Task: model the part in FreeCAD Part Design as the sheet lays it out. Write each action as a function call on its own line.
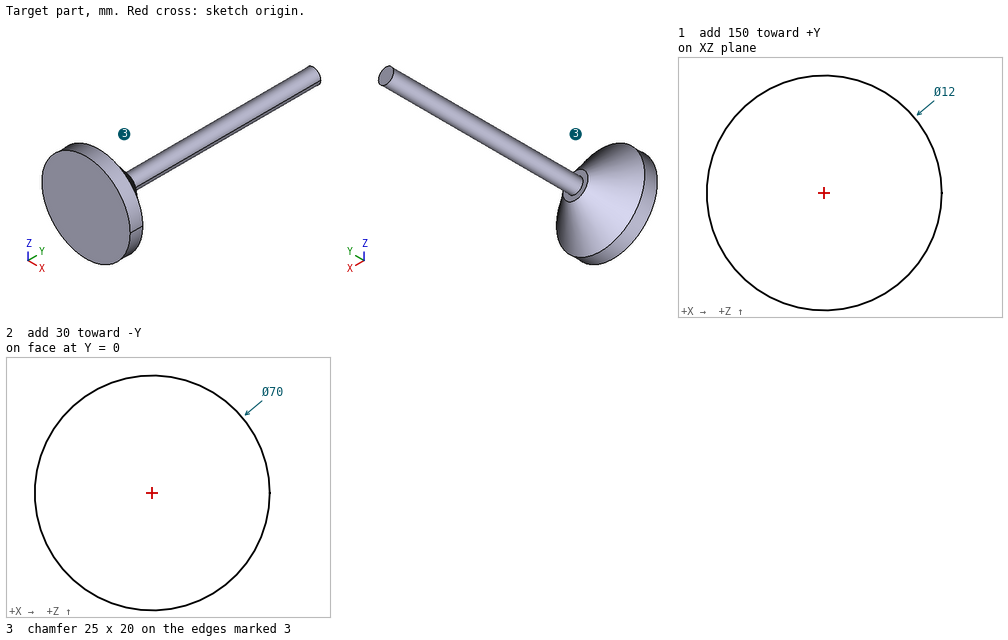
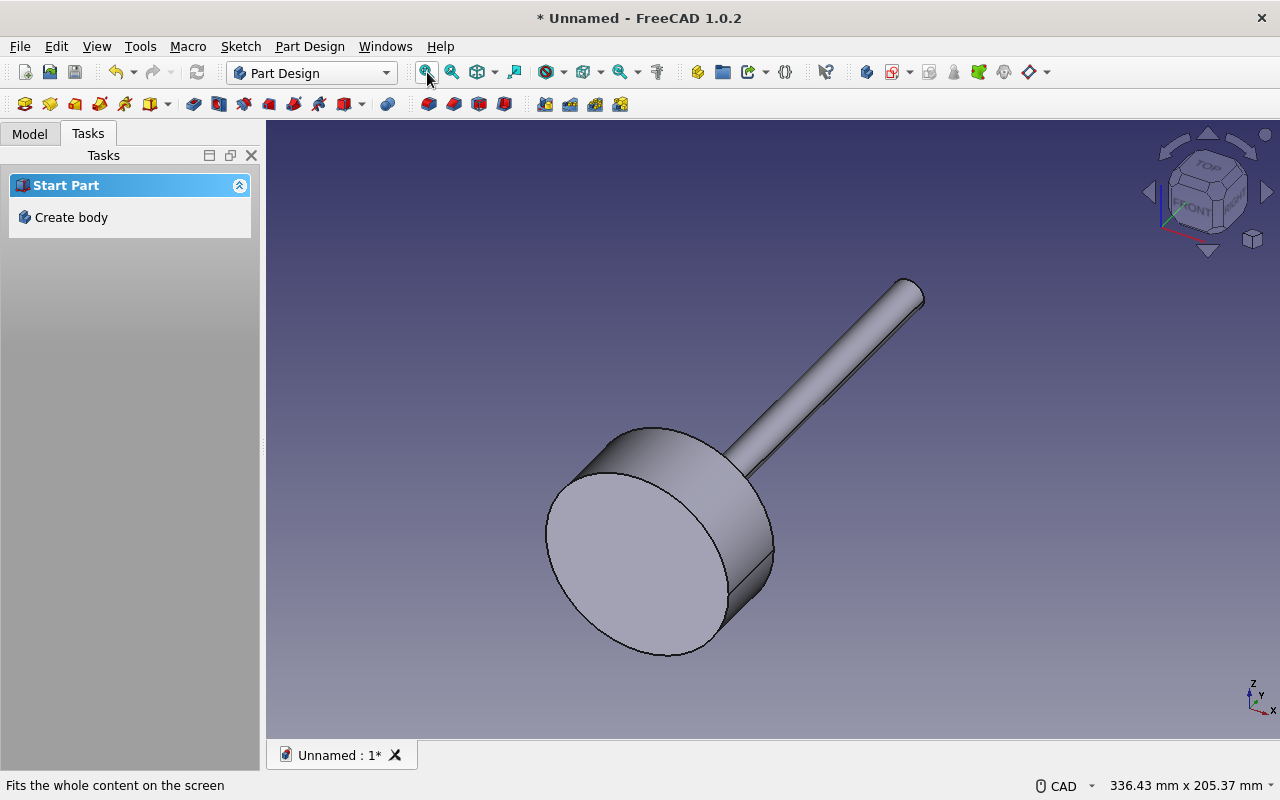
click(711, 445)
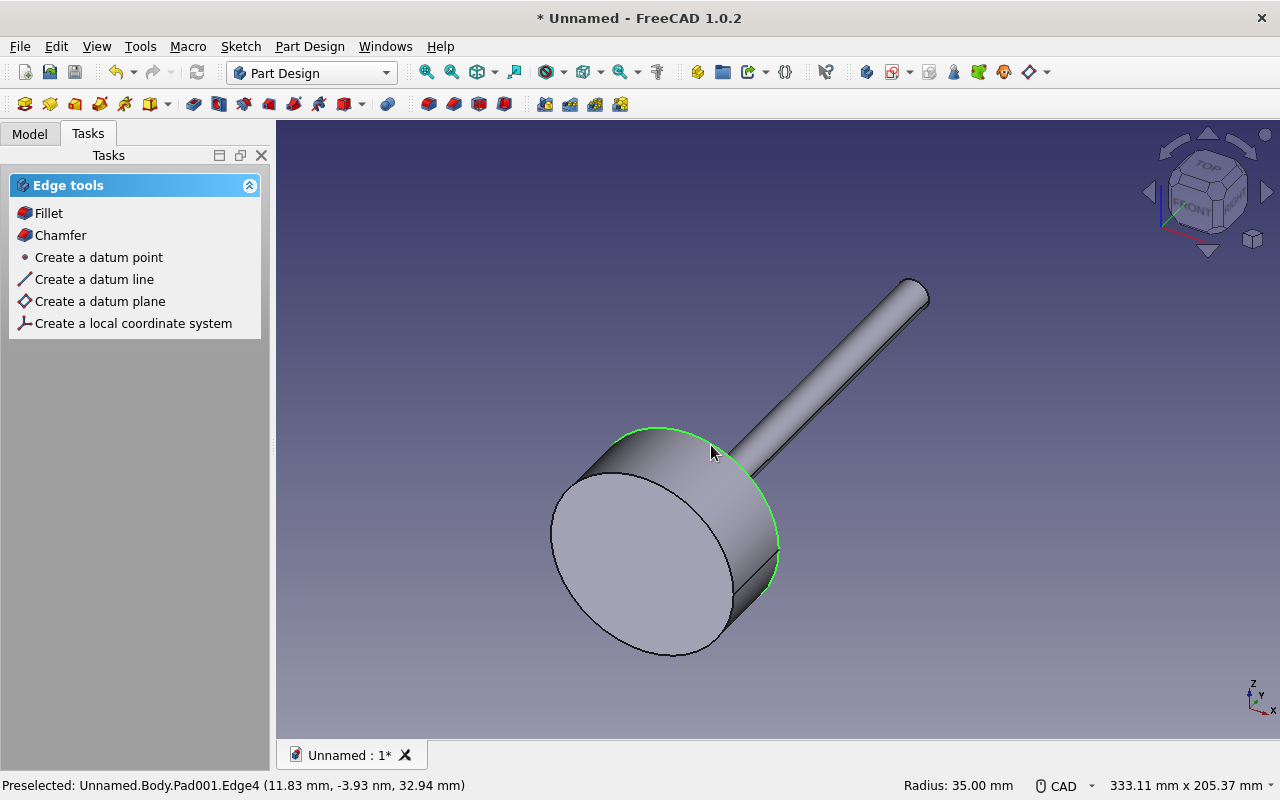
click(454, 104)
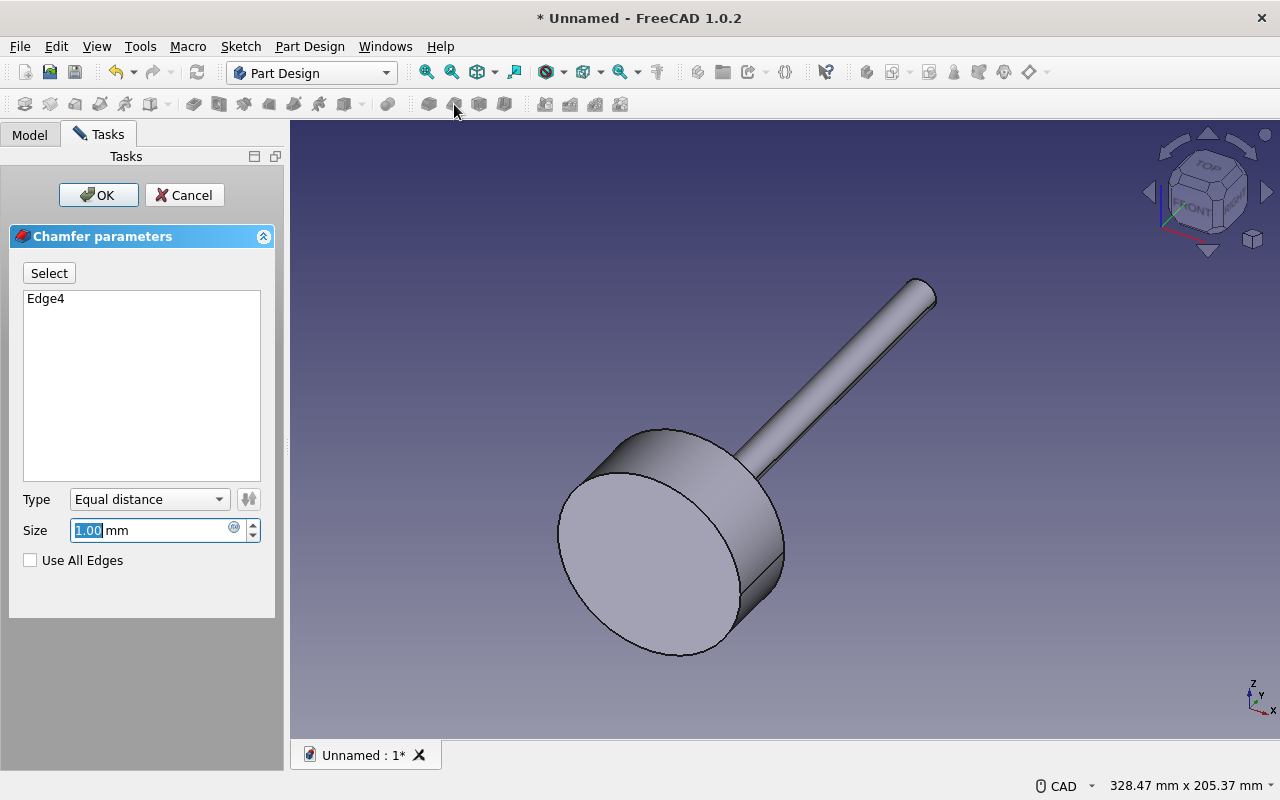
text(25)
key(Tab)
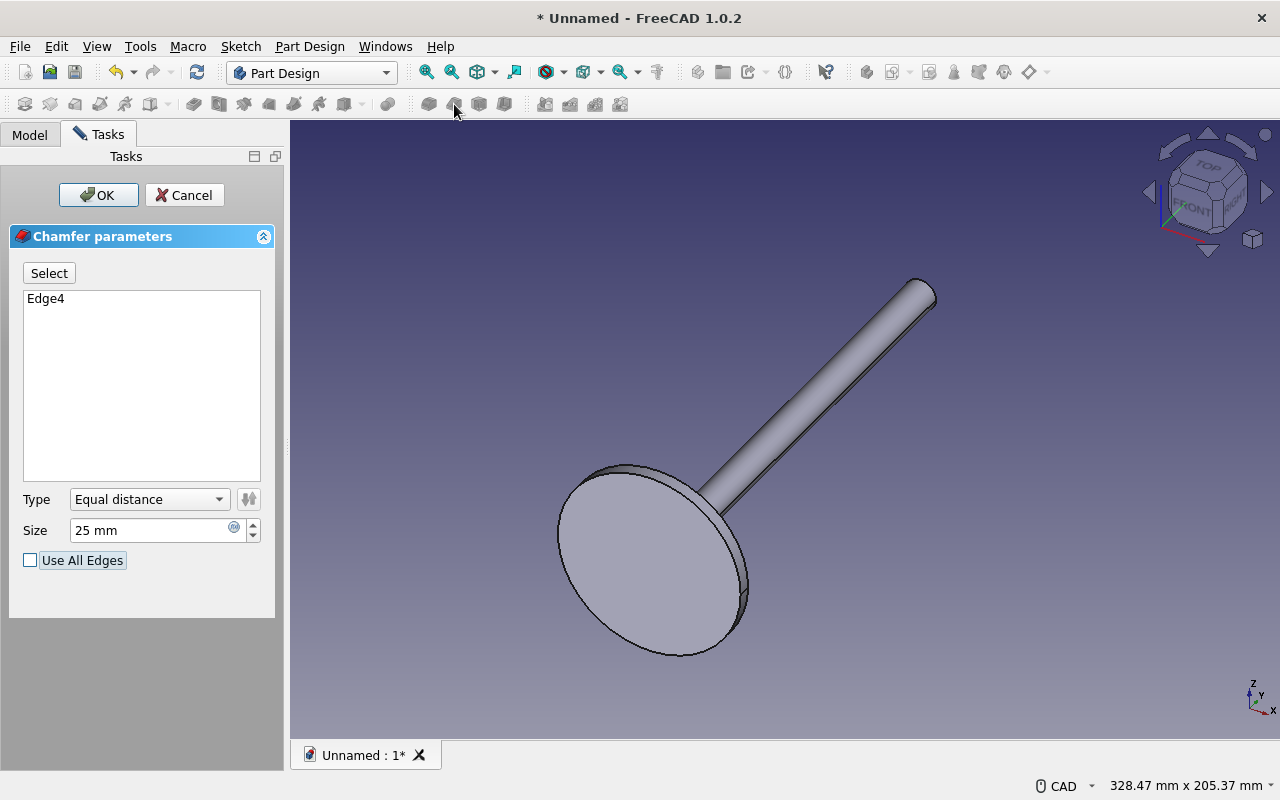
click(150, 500)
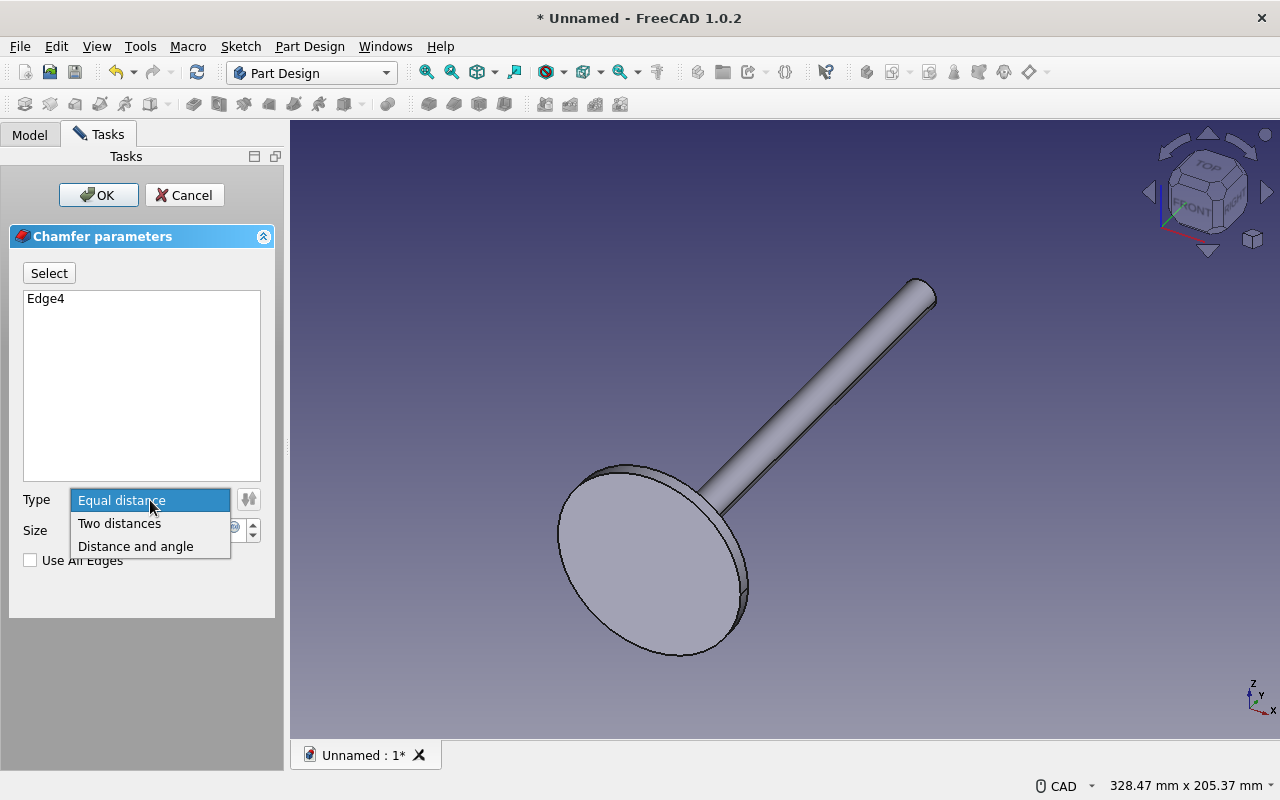
click(148, 524)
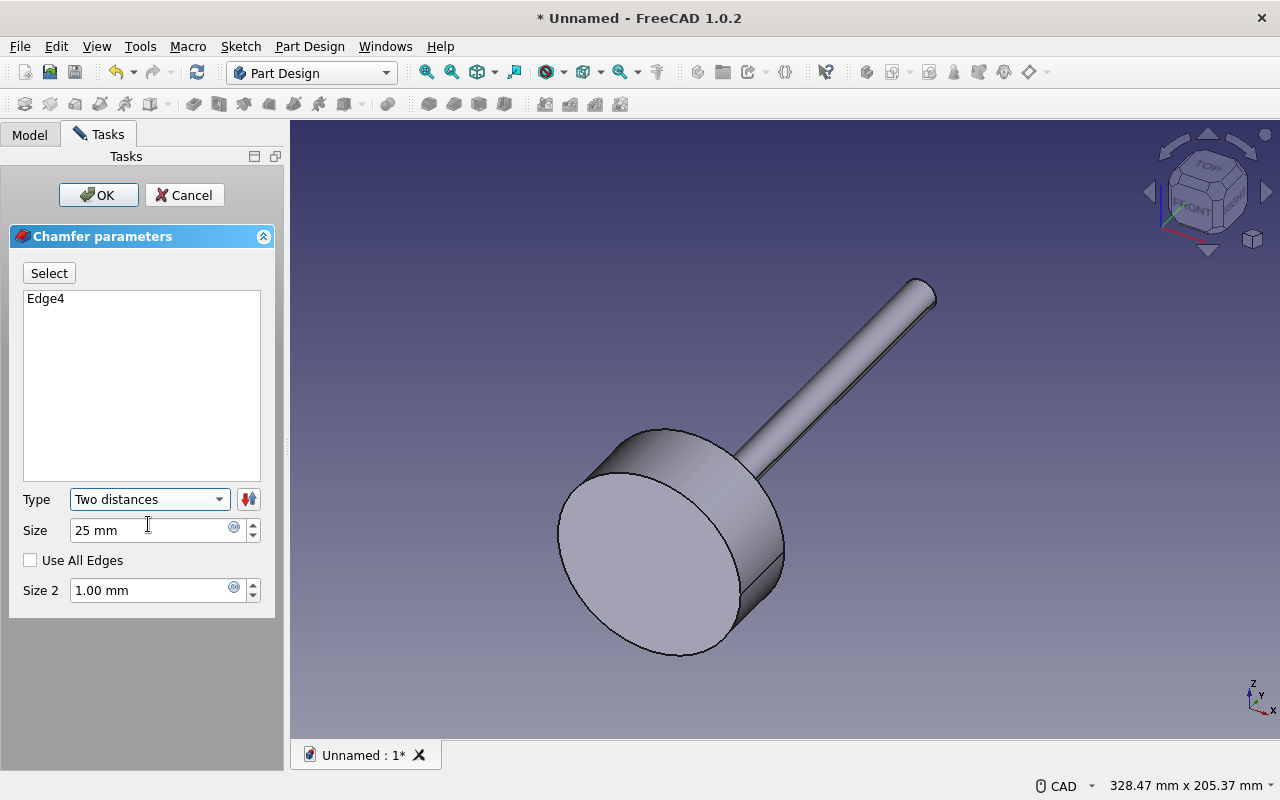
triple_click(158, 590)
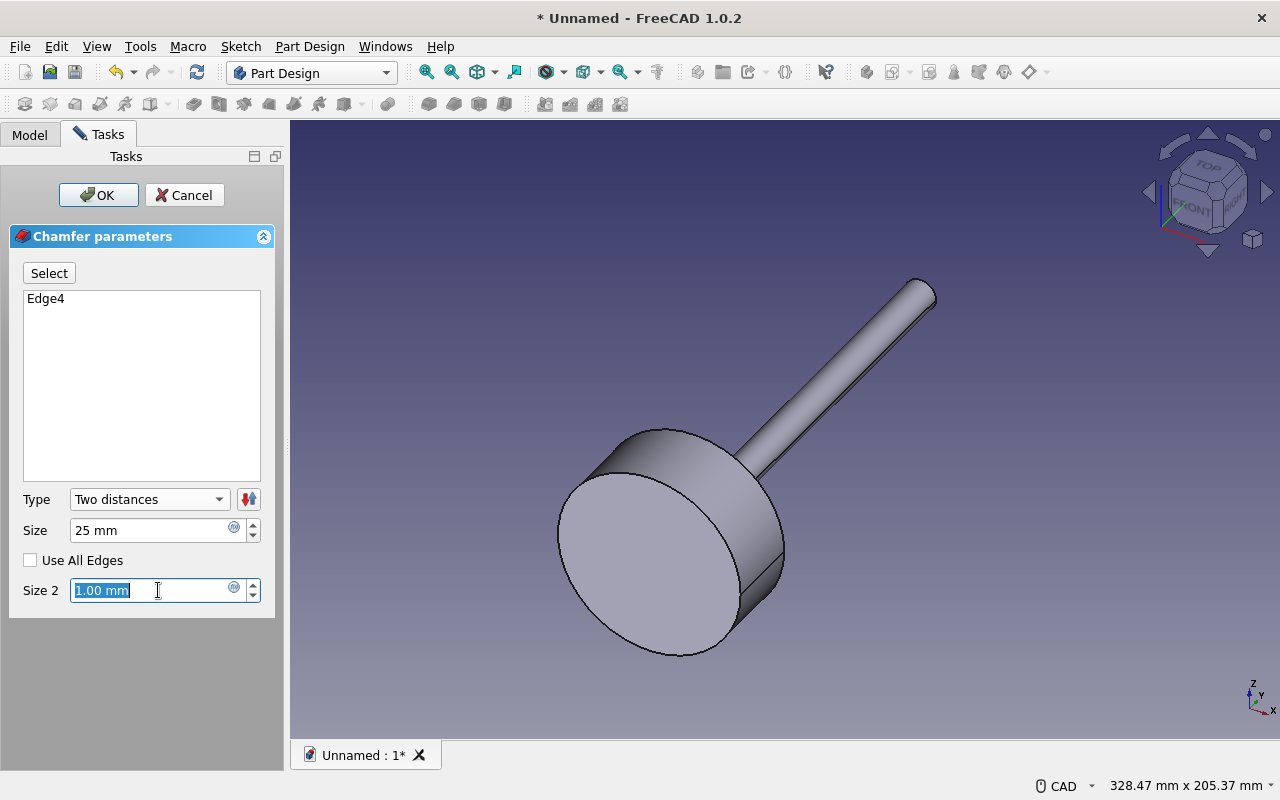
text(20)
key(Tab)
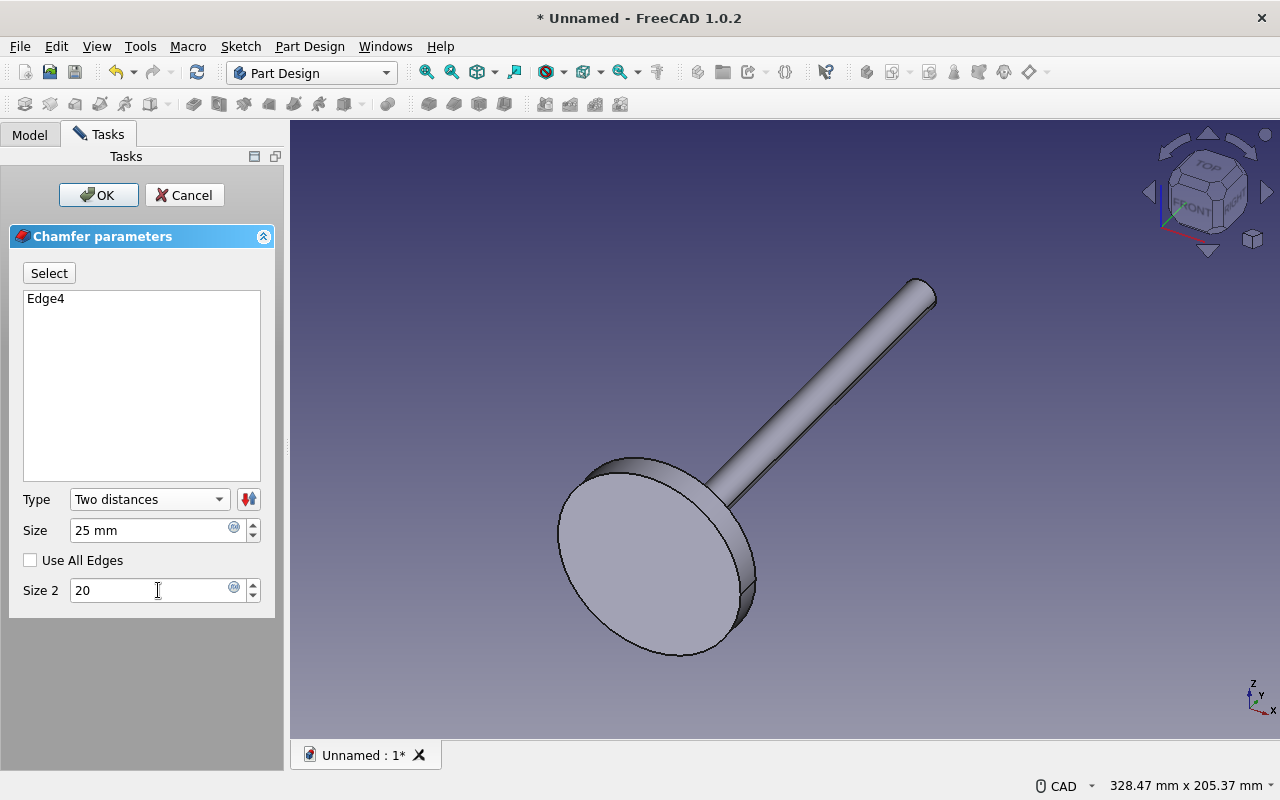
click(99, 195)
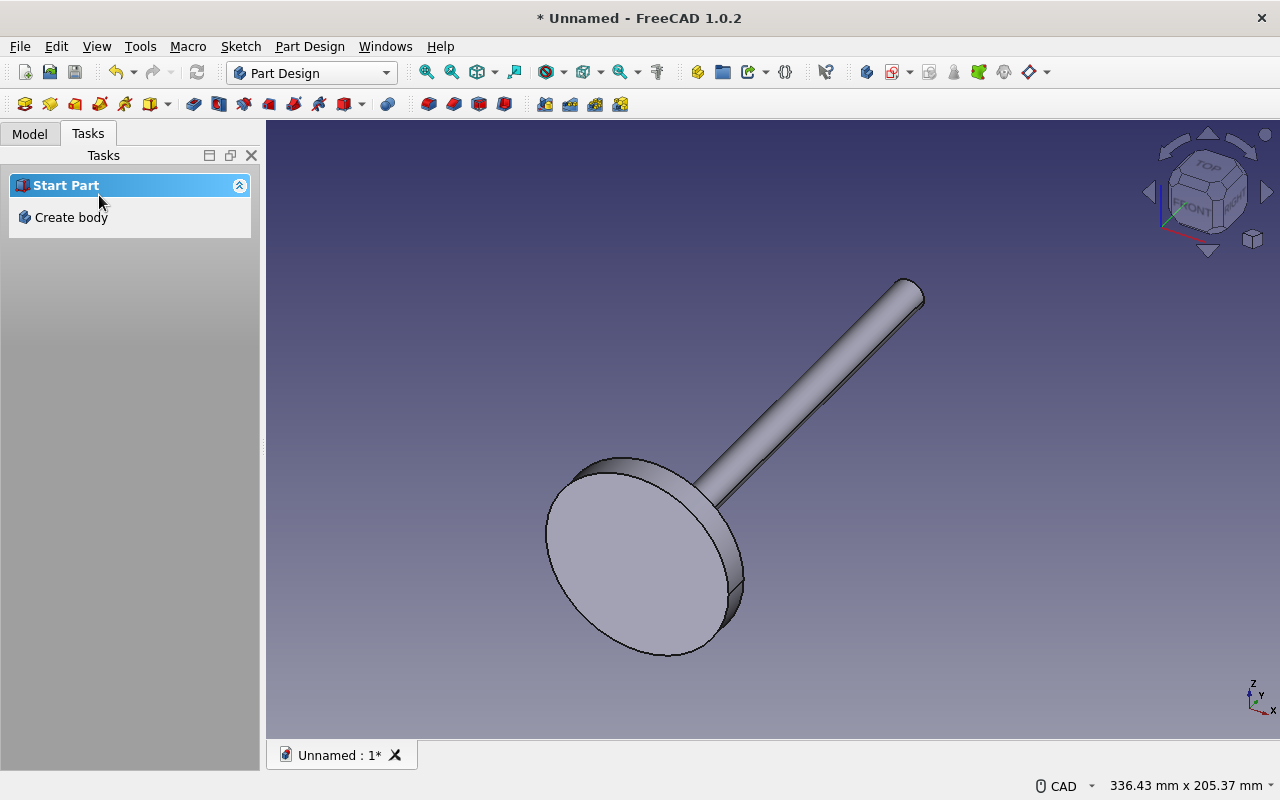
key(0)